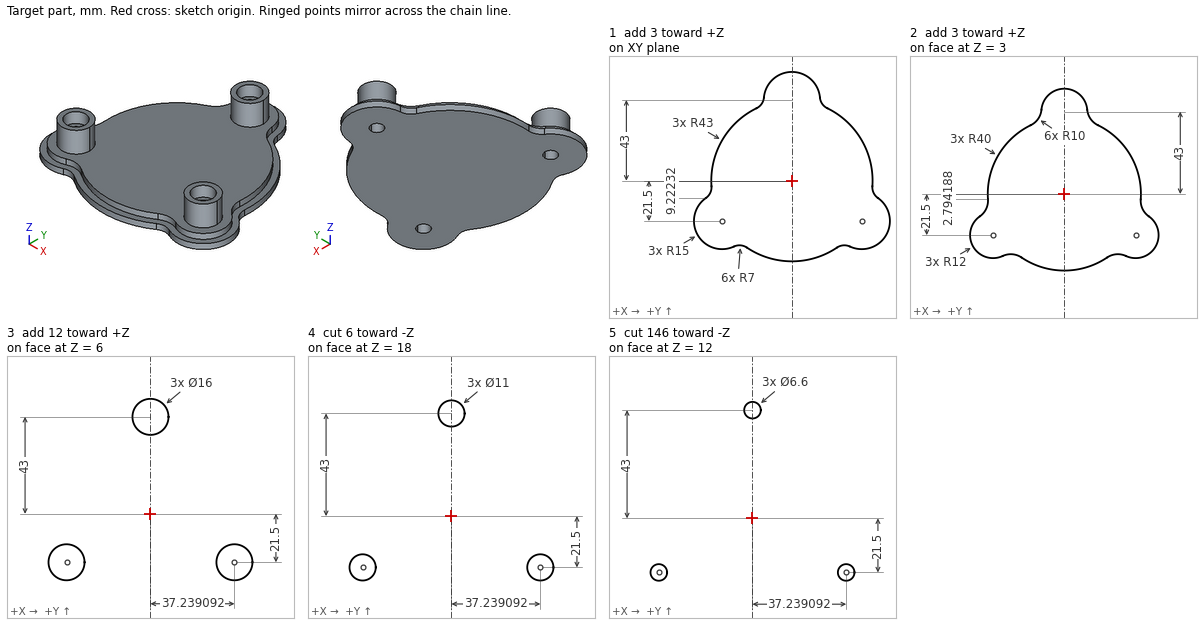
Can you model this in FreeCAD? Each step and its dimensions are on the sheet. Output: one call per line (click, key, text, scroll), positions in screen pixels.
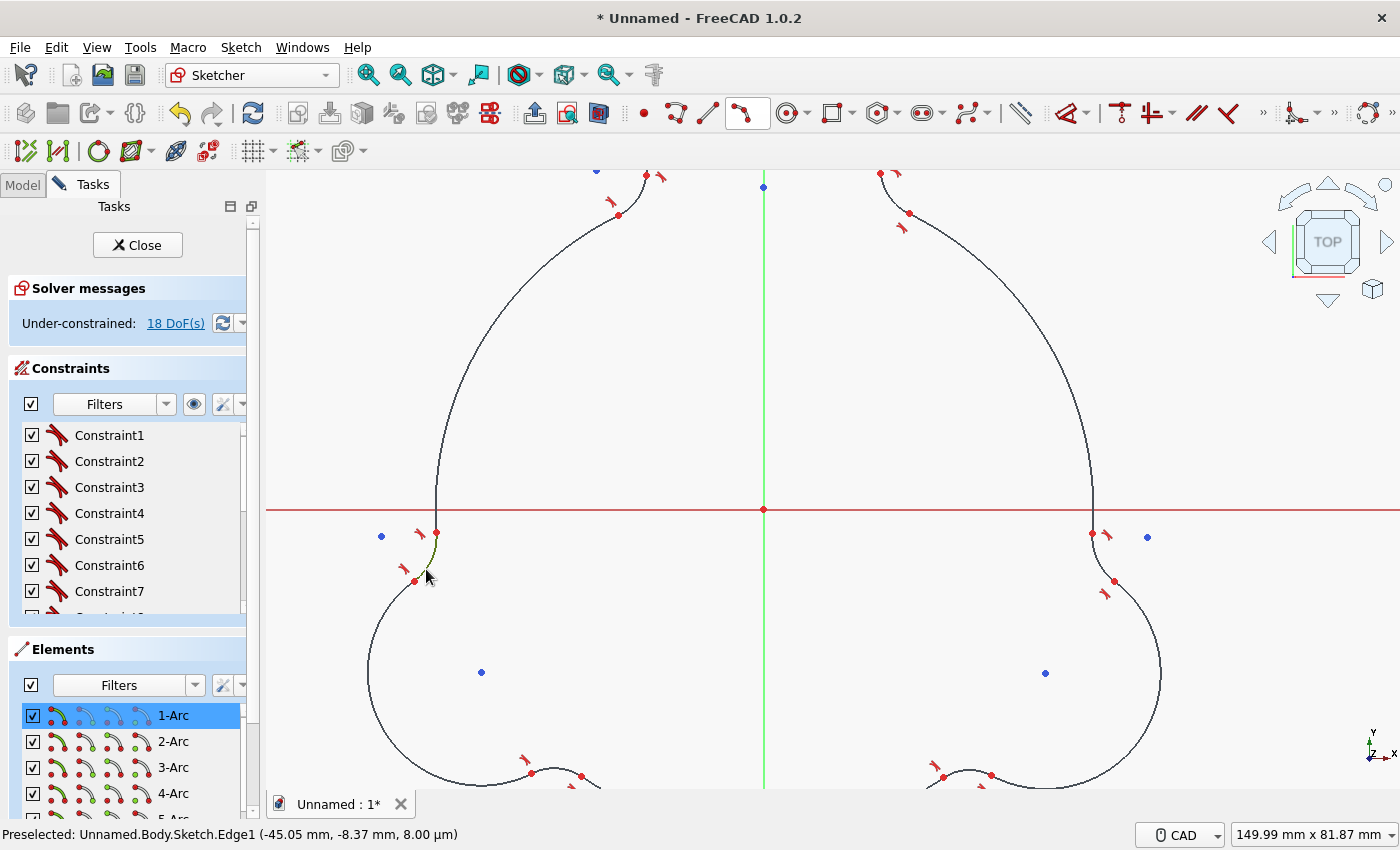
scroll(766, 512, down, 3)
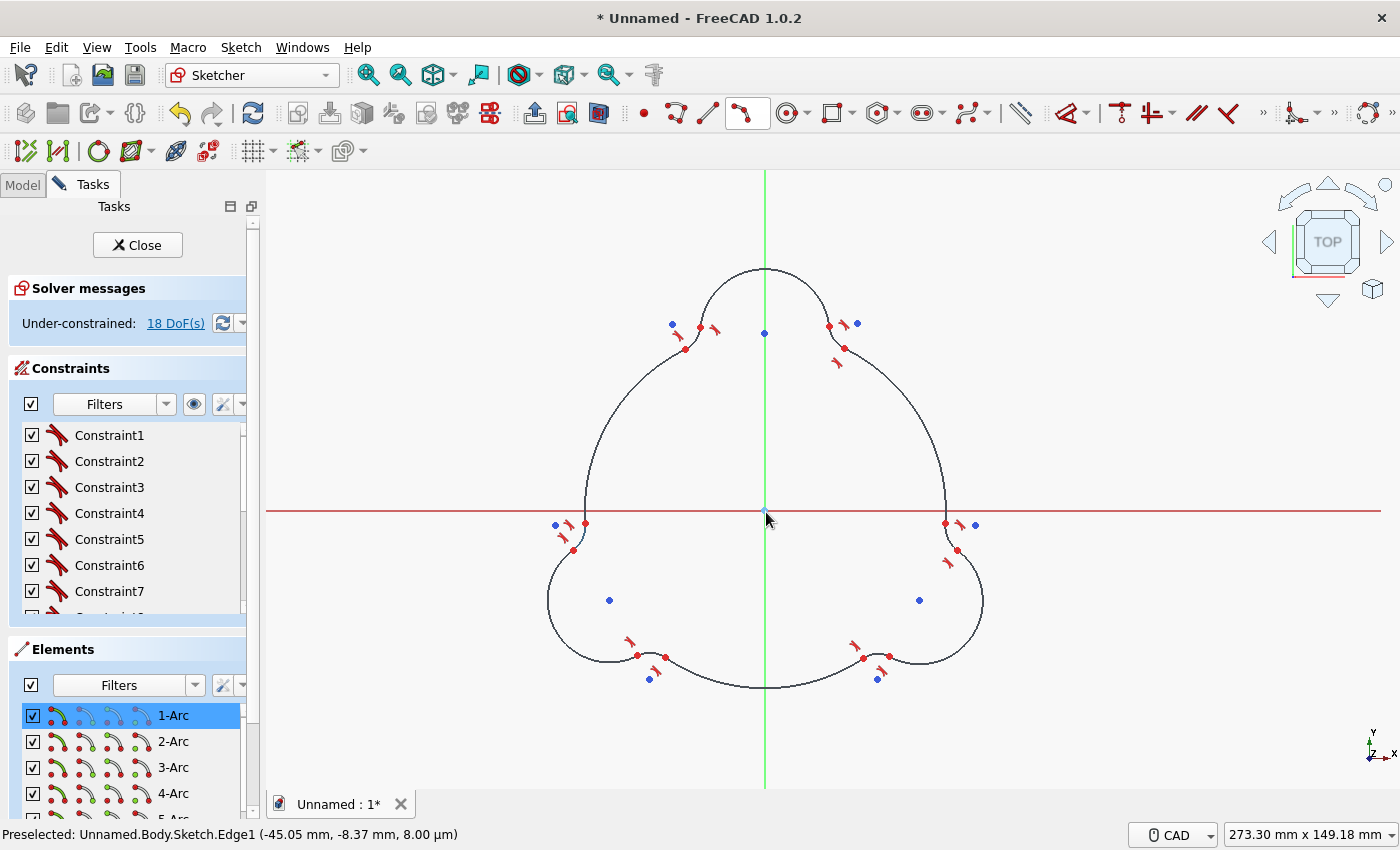
scroll(657, 654, up, 3)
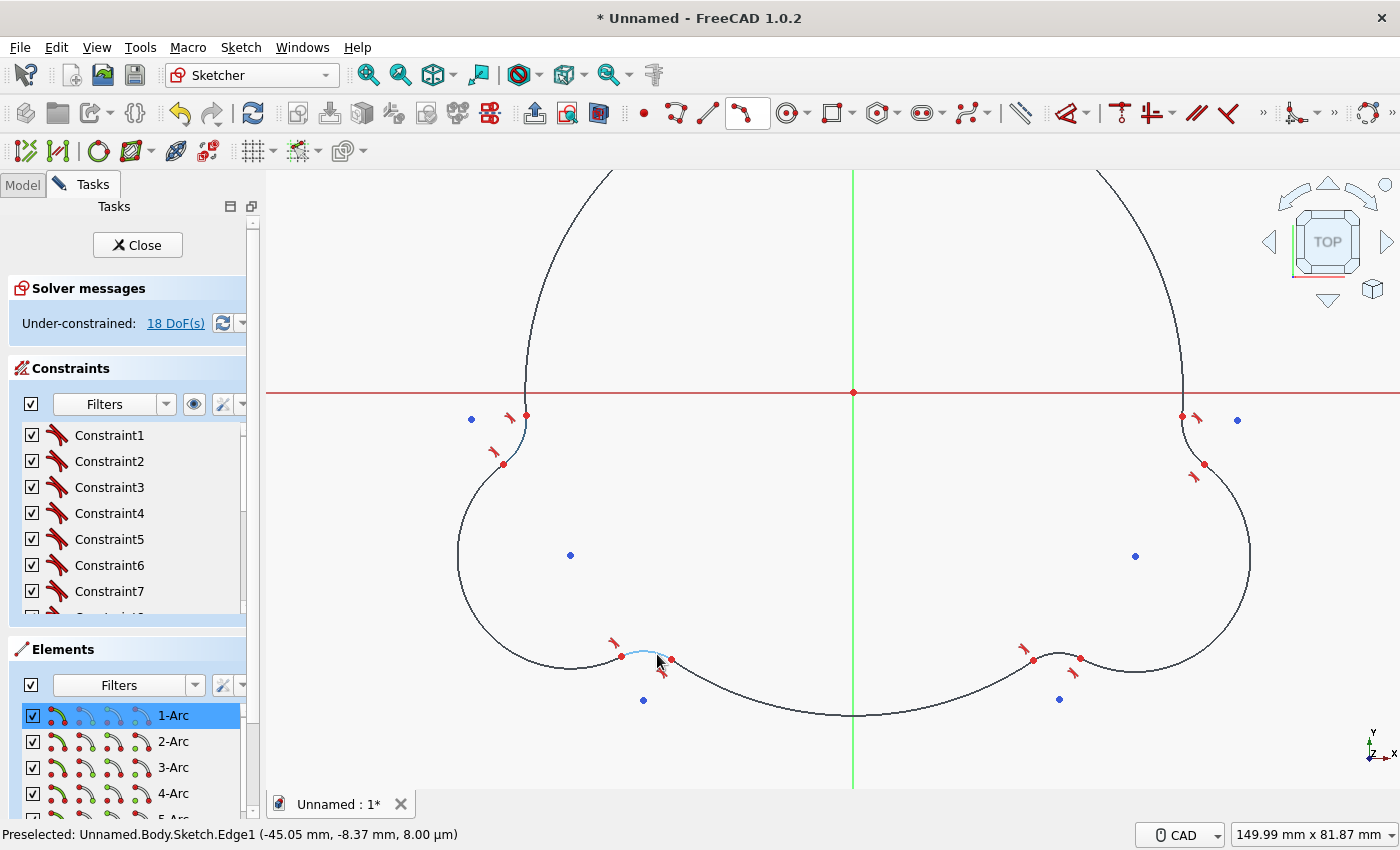
click(657, 653)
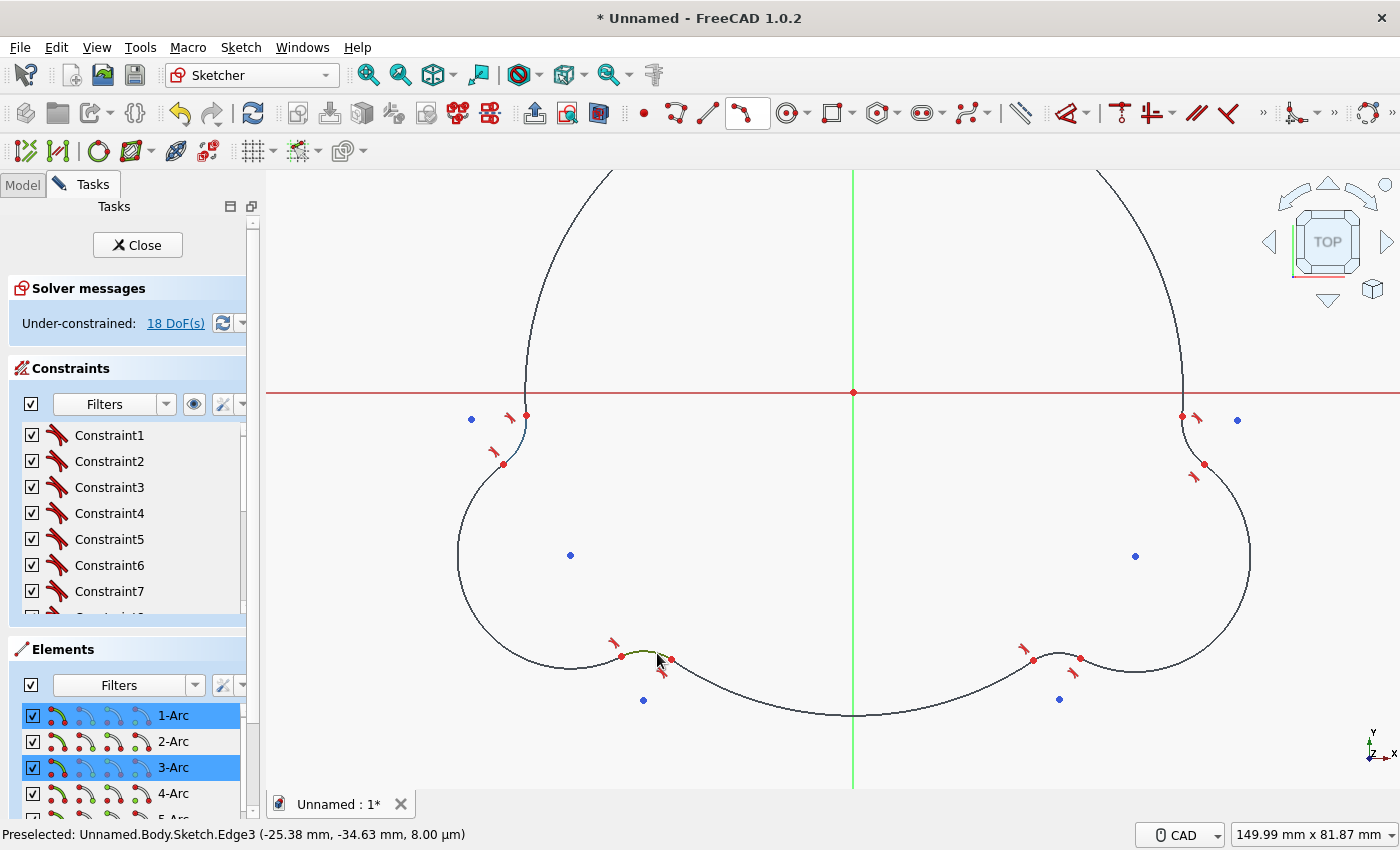
click(1067, 654)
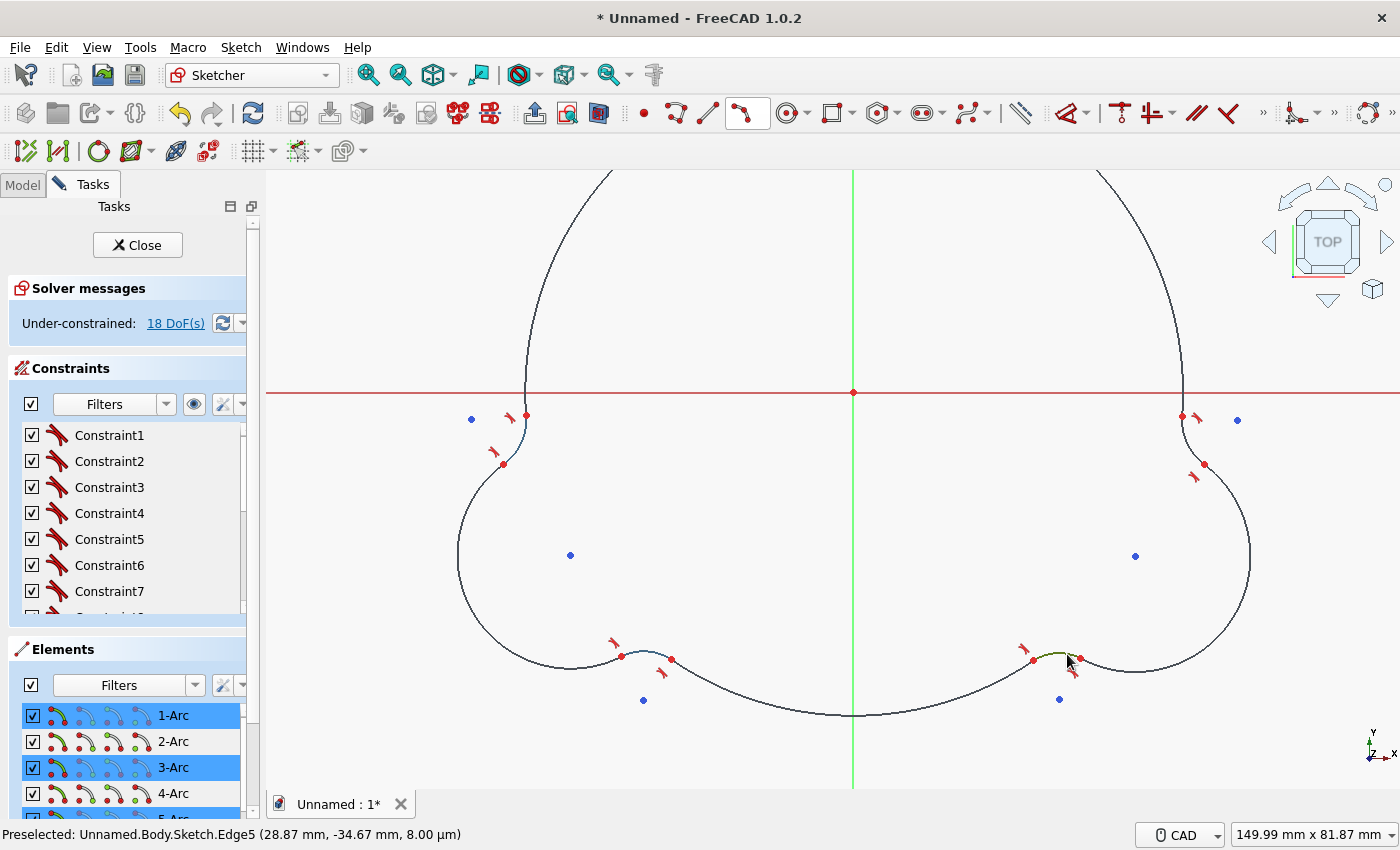
click(1184, 433)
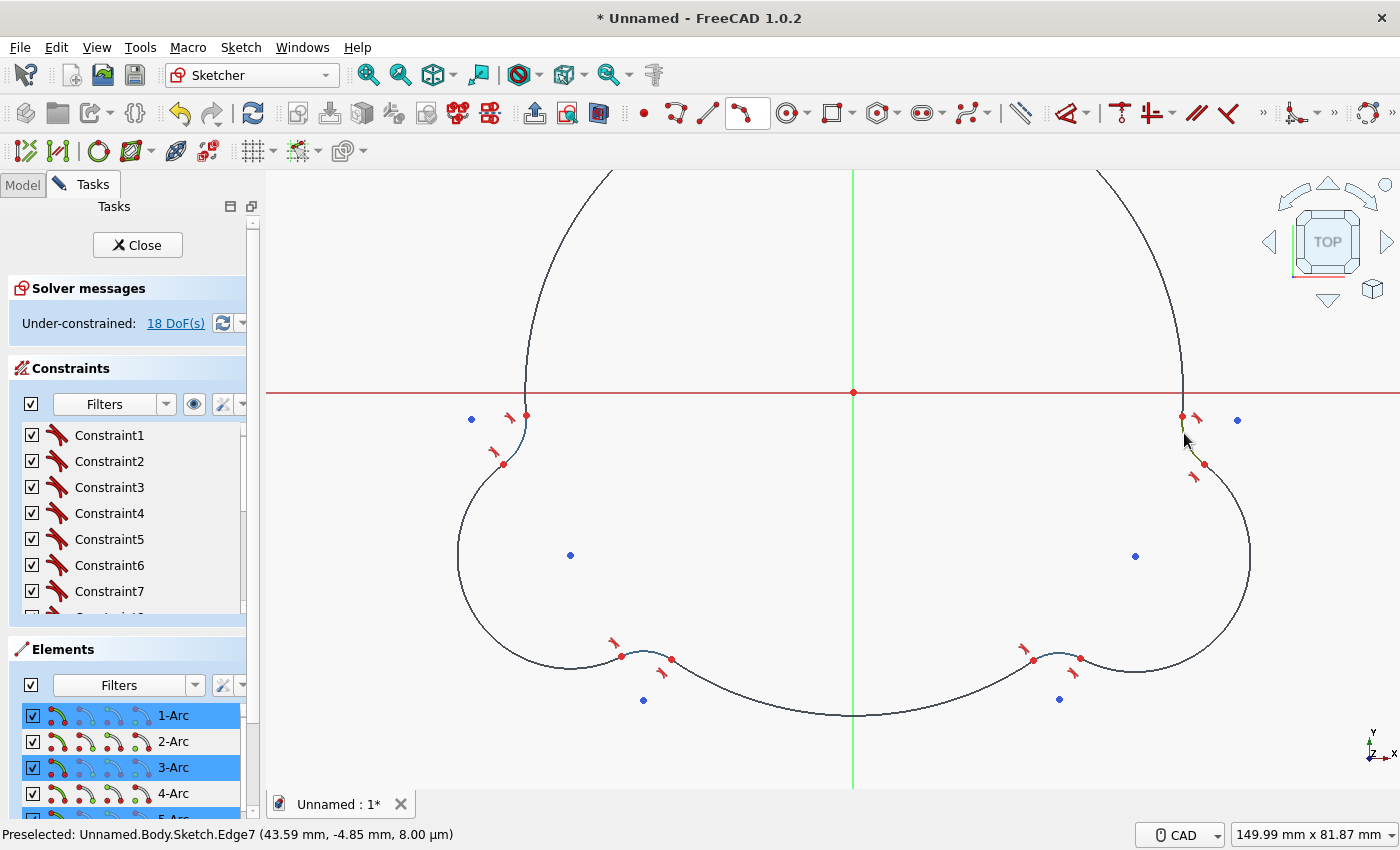
scroll(656, 654, down, 3)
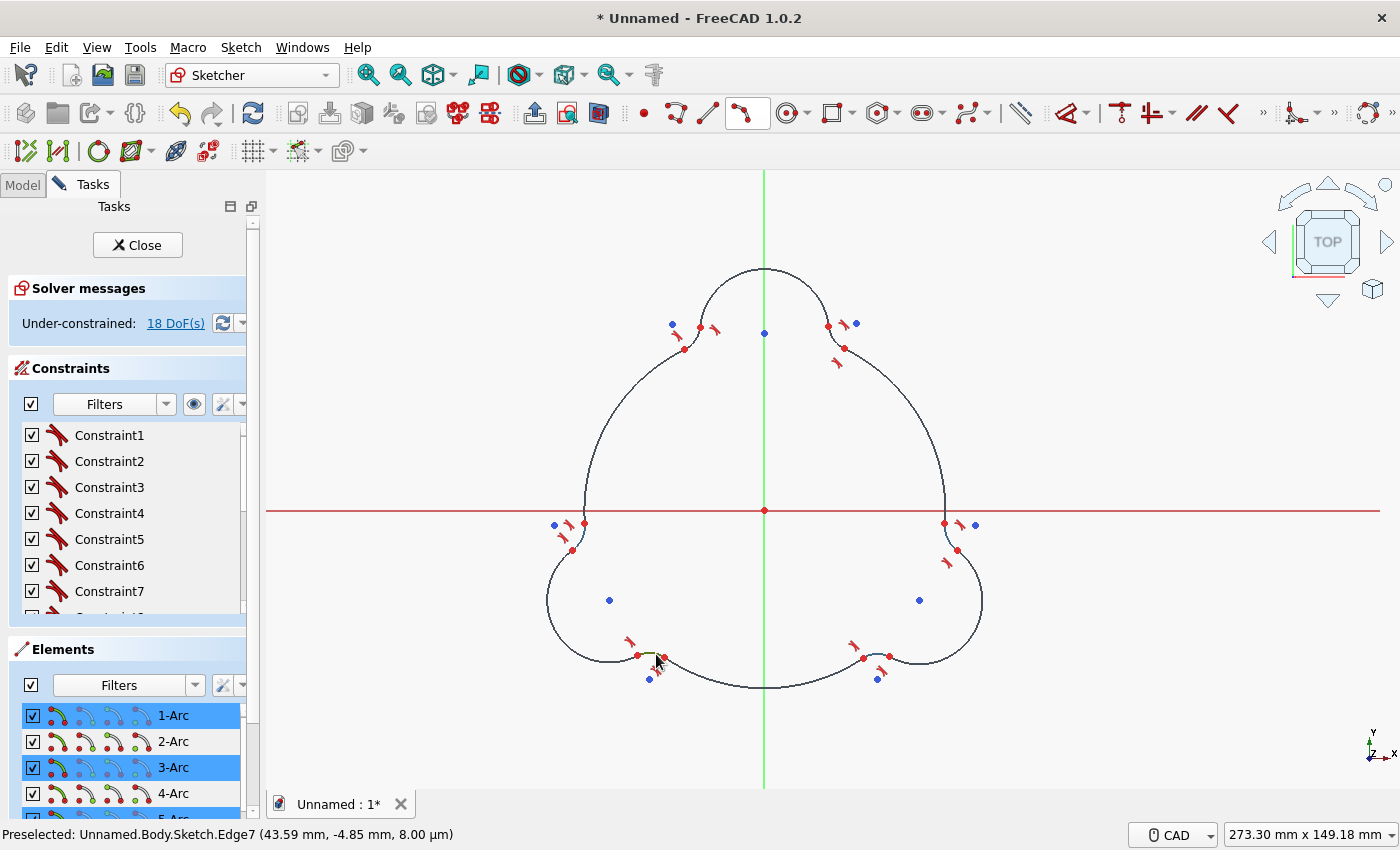
scroll(831, 335, up, 3)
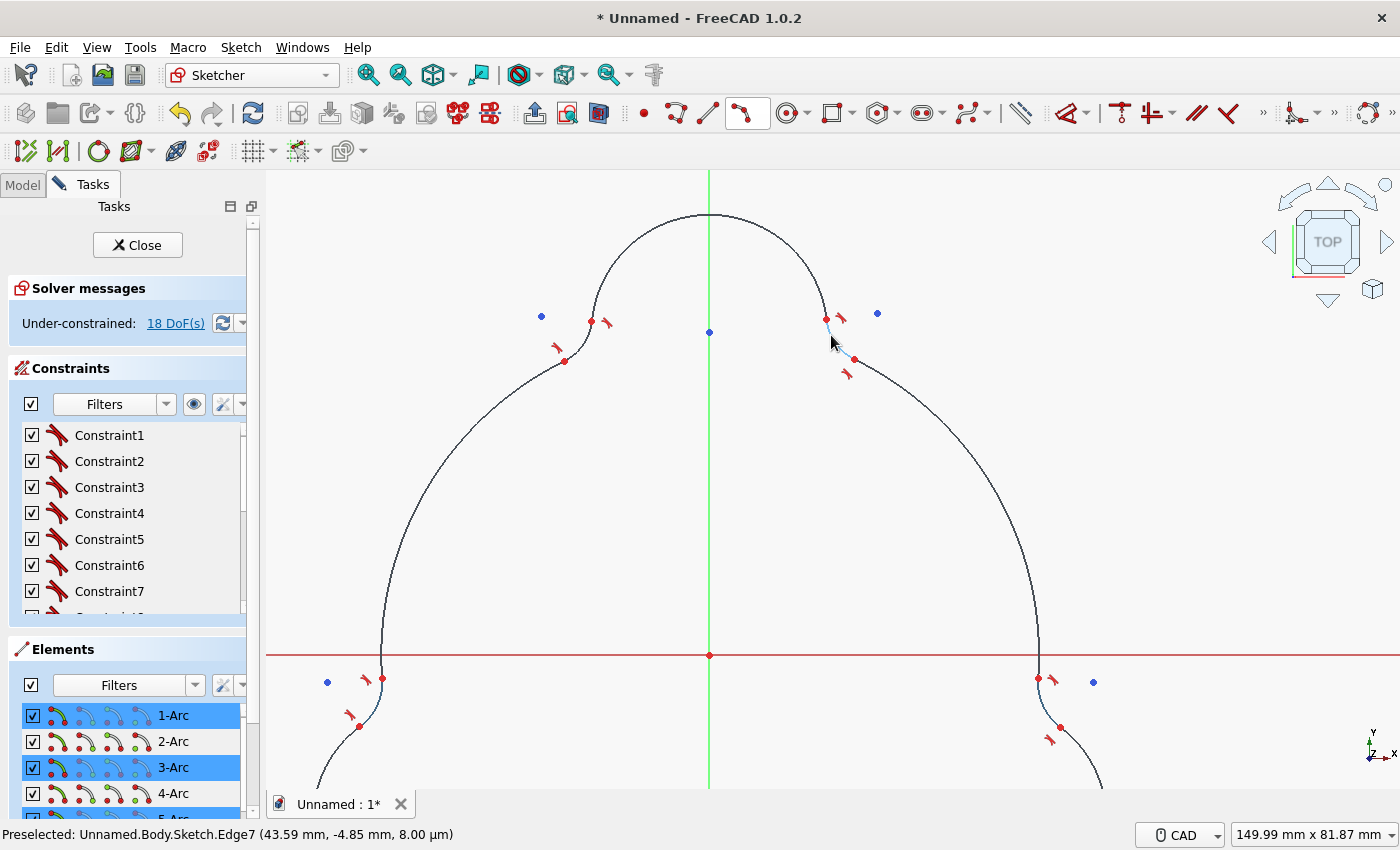
click(831, 334)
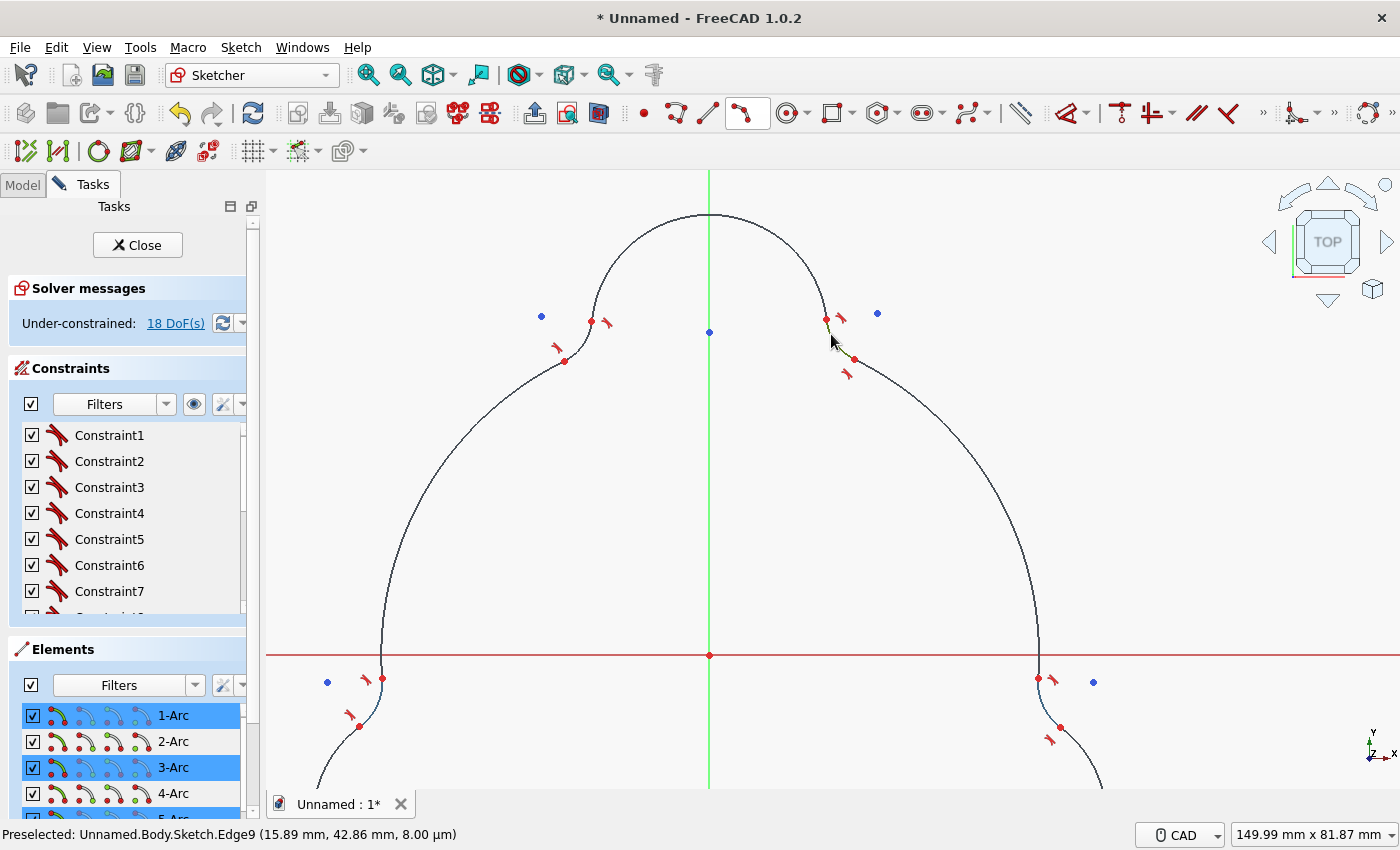
click(577, 353)